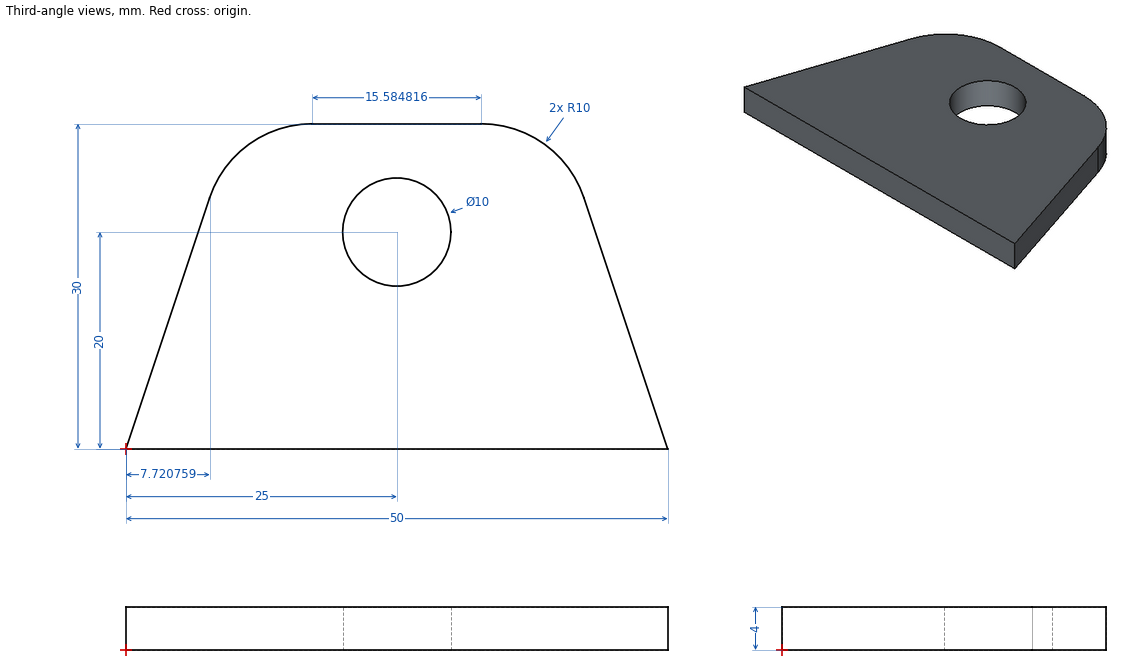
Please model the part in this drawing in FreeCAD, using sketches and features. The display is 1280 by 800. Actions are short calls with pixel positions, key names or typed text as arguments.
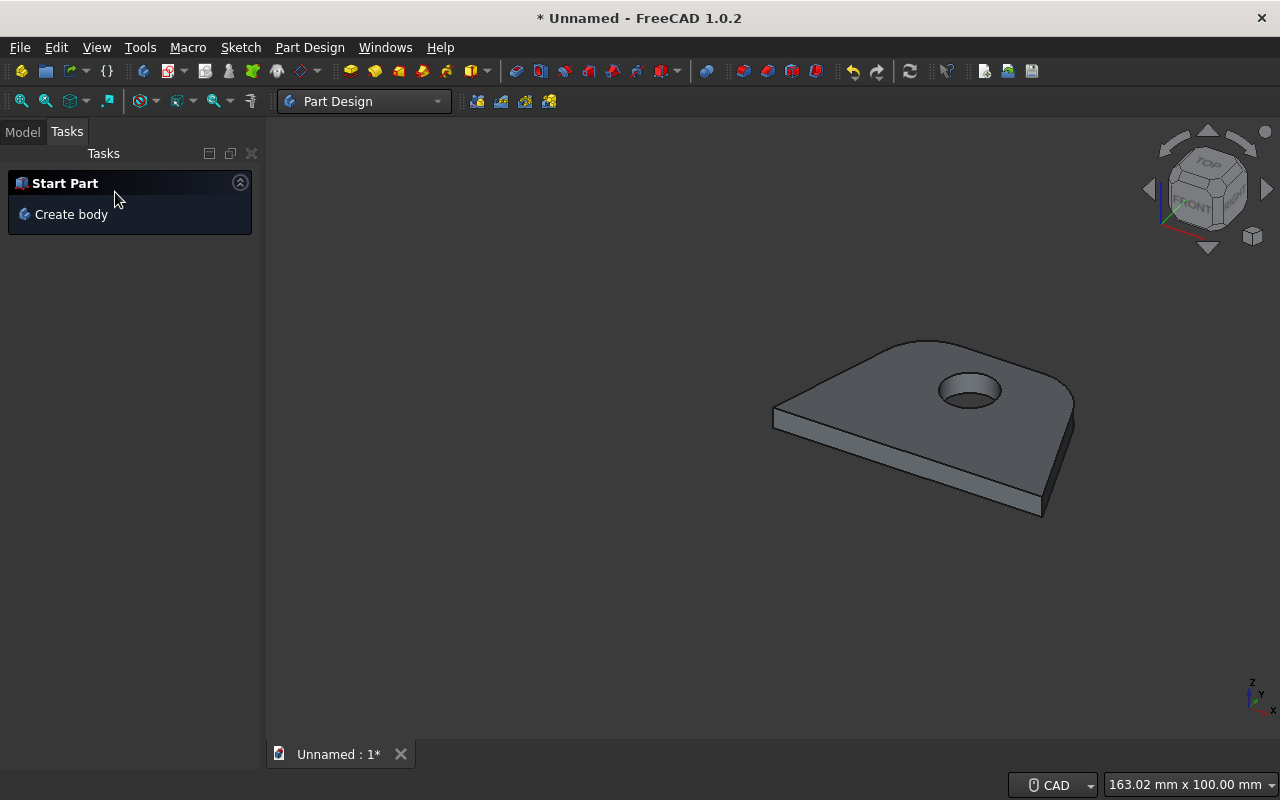
key(0)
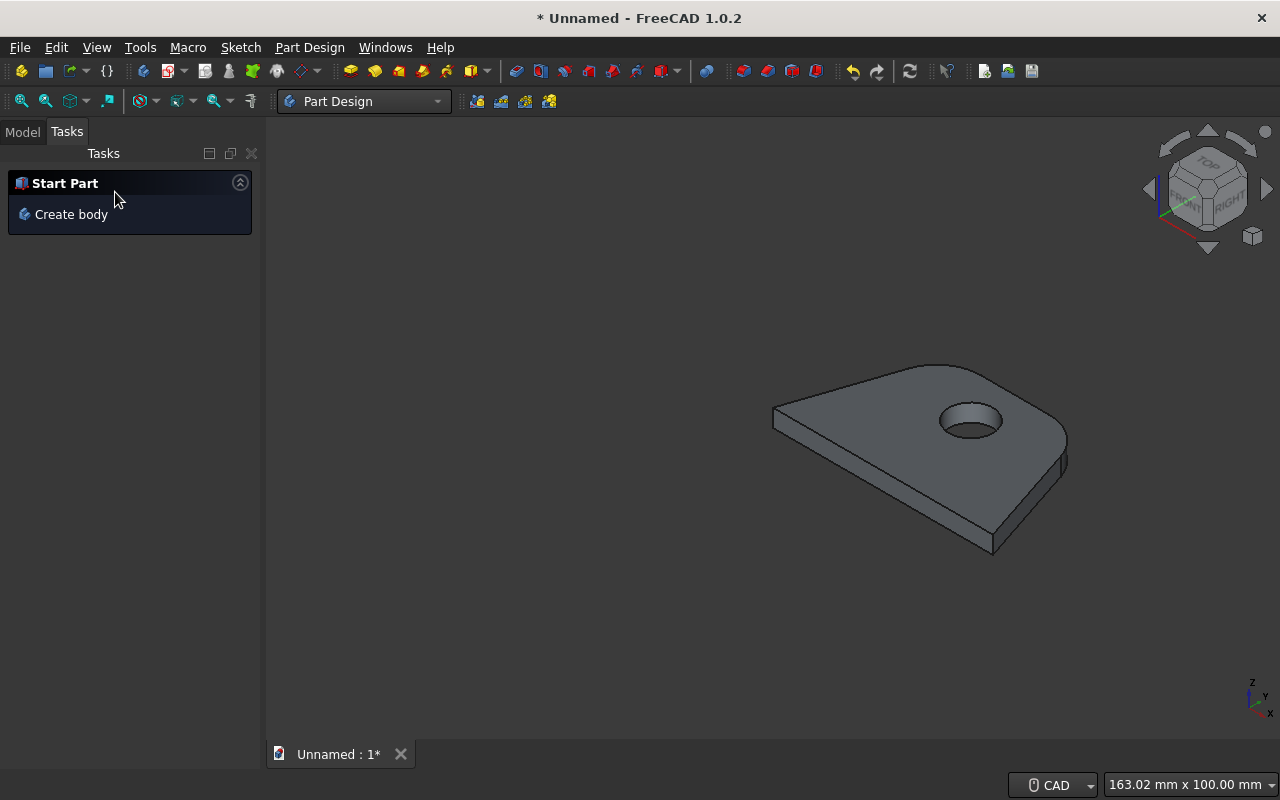
click(22, 102)